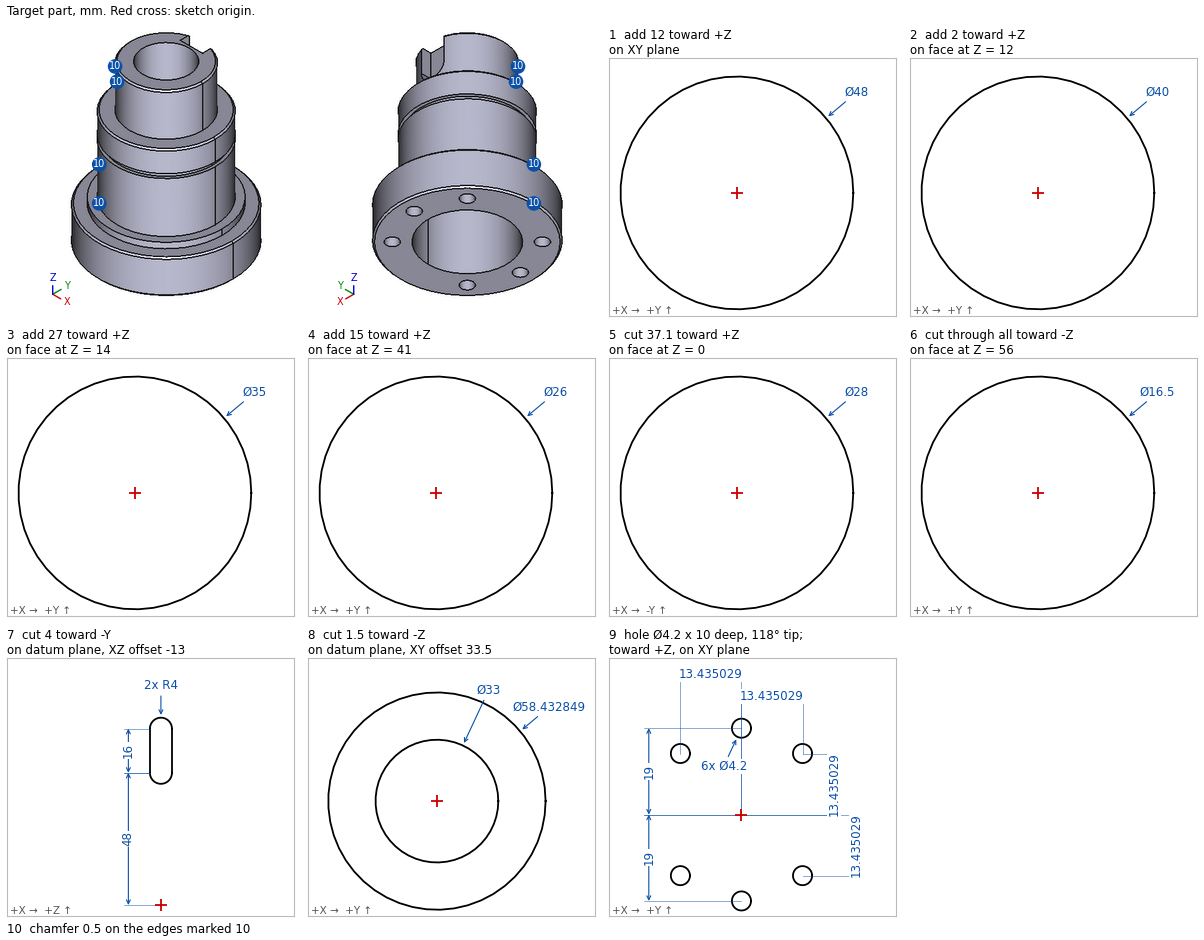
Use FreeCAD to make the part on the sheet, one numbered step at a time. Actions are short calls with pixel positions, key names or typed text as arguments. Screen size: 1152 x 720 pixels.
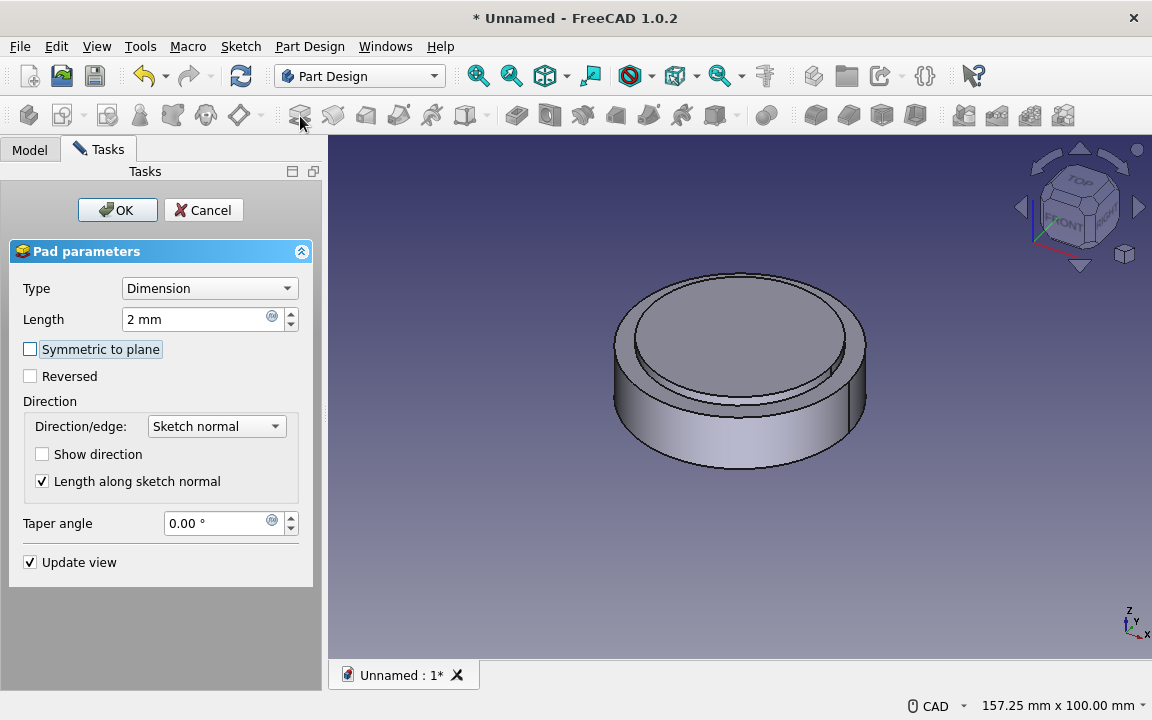
click(118, 210)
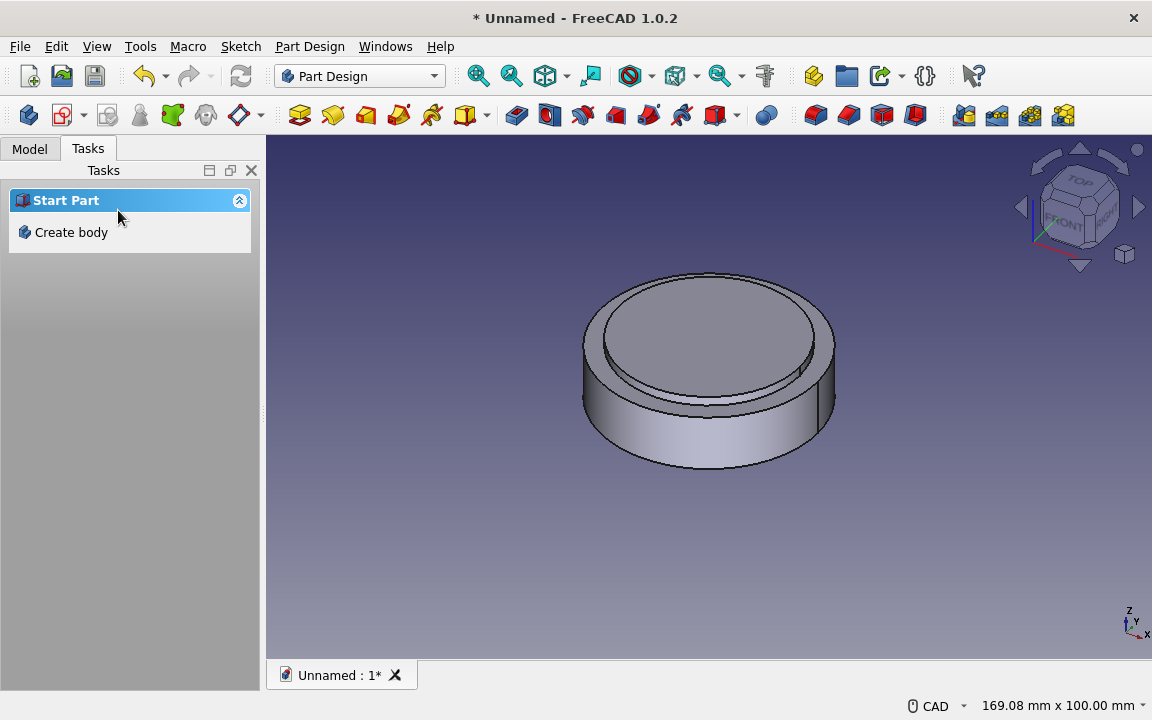
click(709, 336)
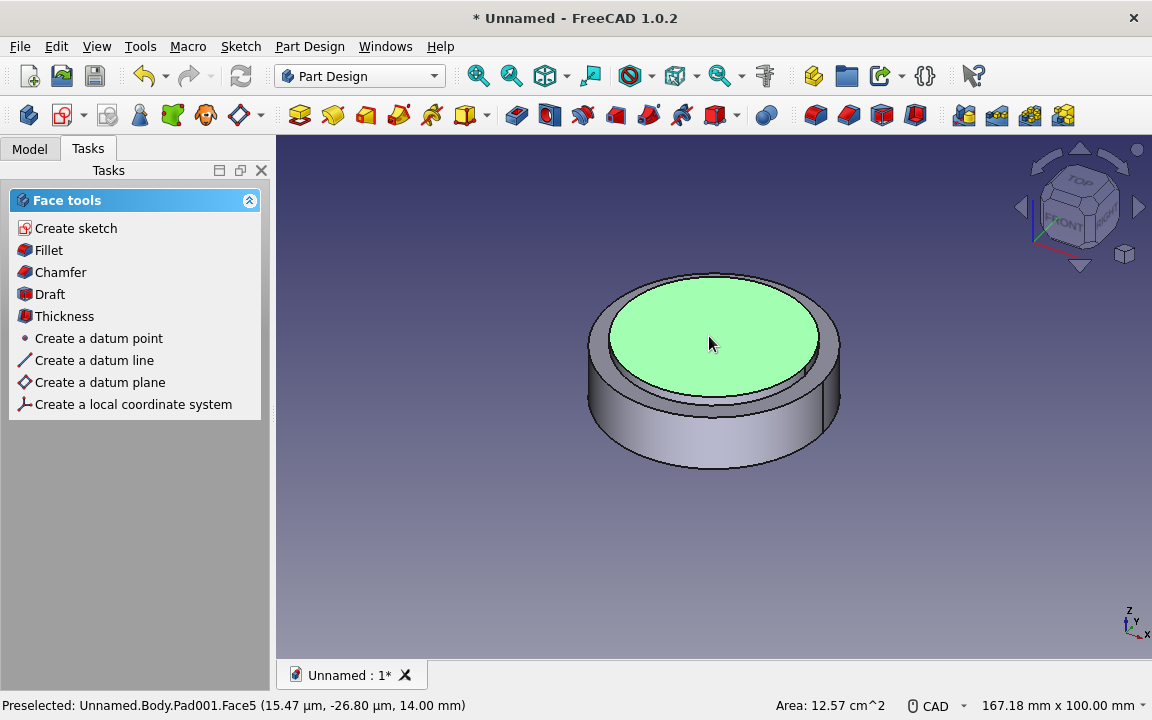
click(62, 116)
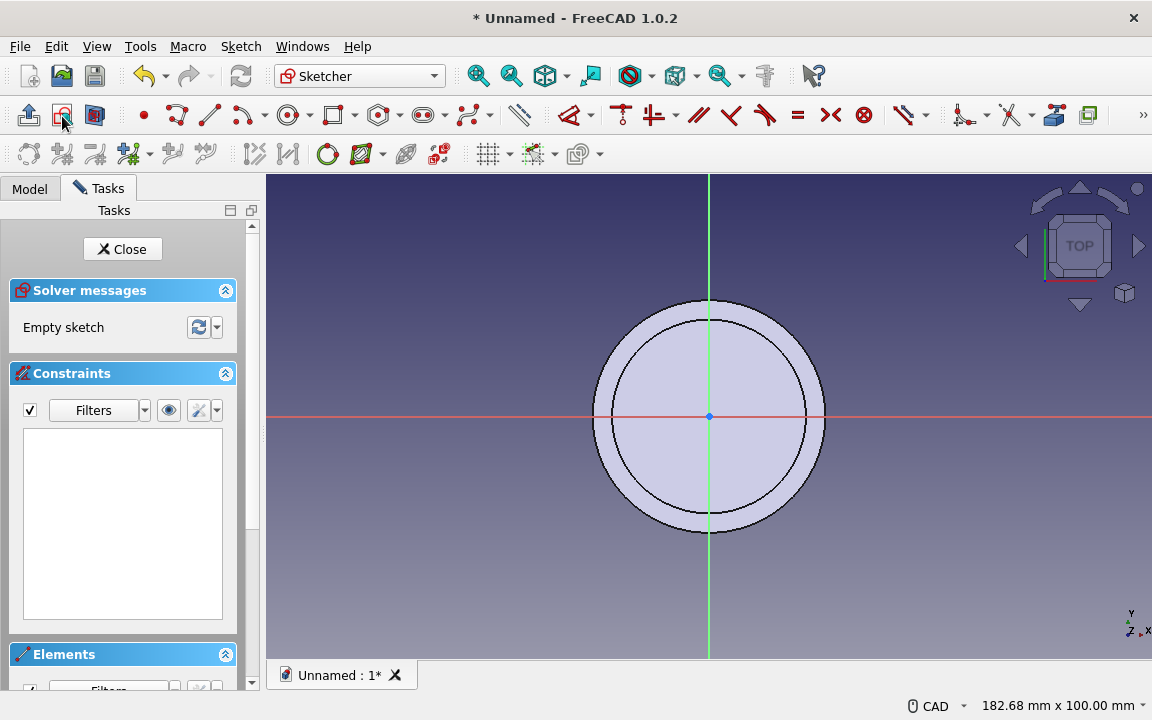
scroll(792, 416, up, 3)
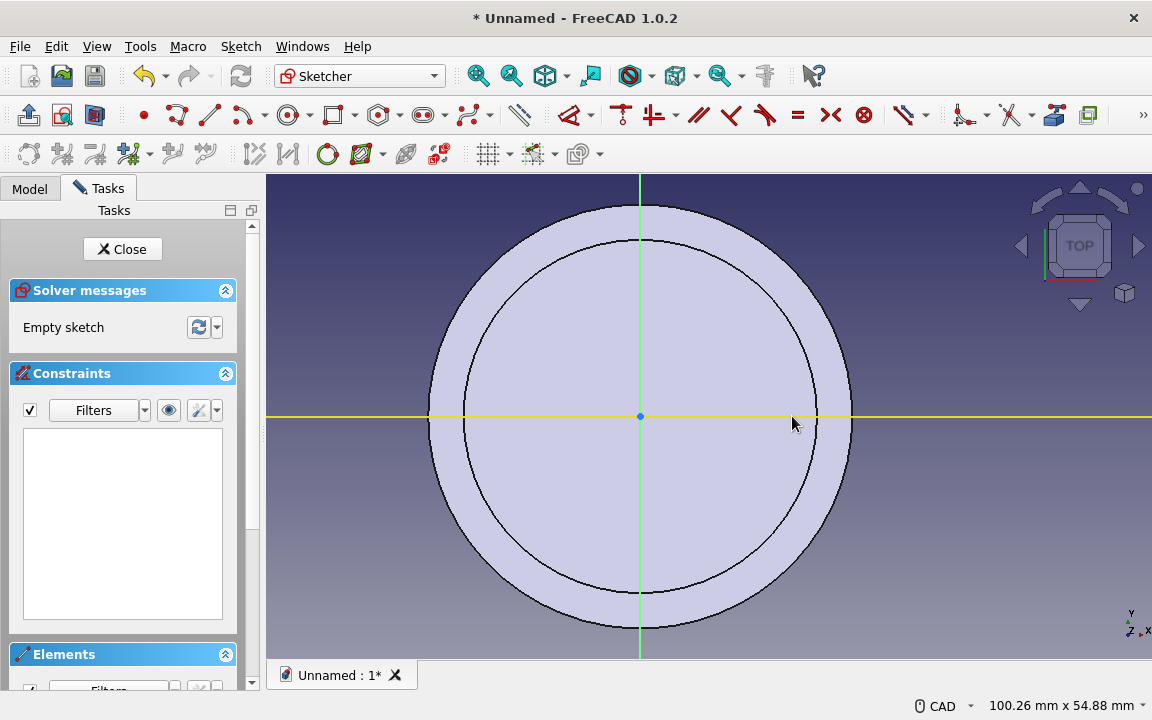
click(288, 116)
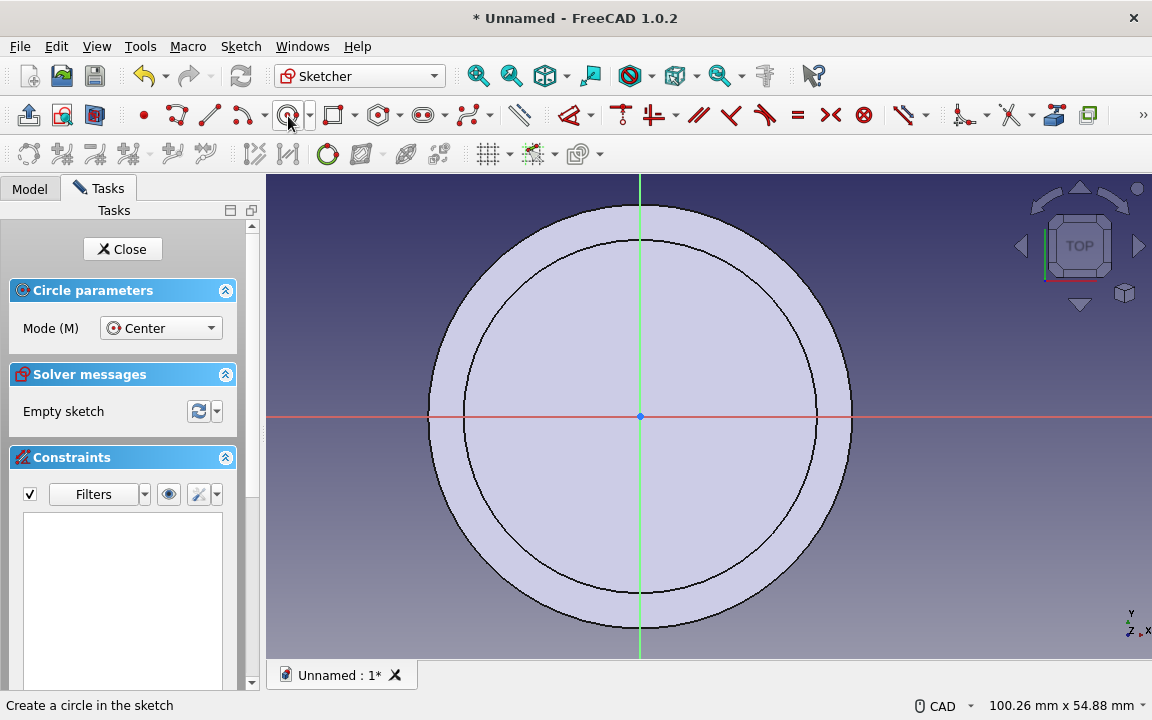
click(640, 416)
click(750, 307)
key(Escape)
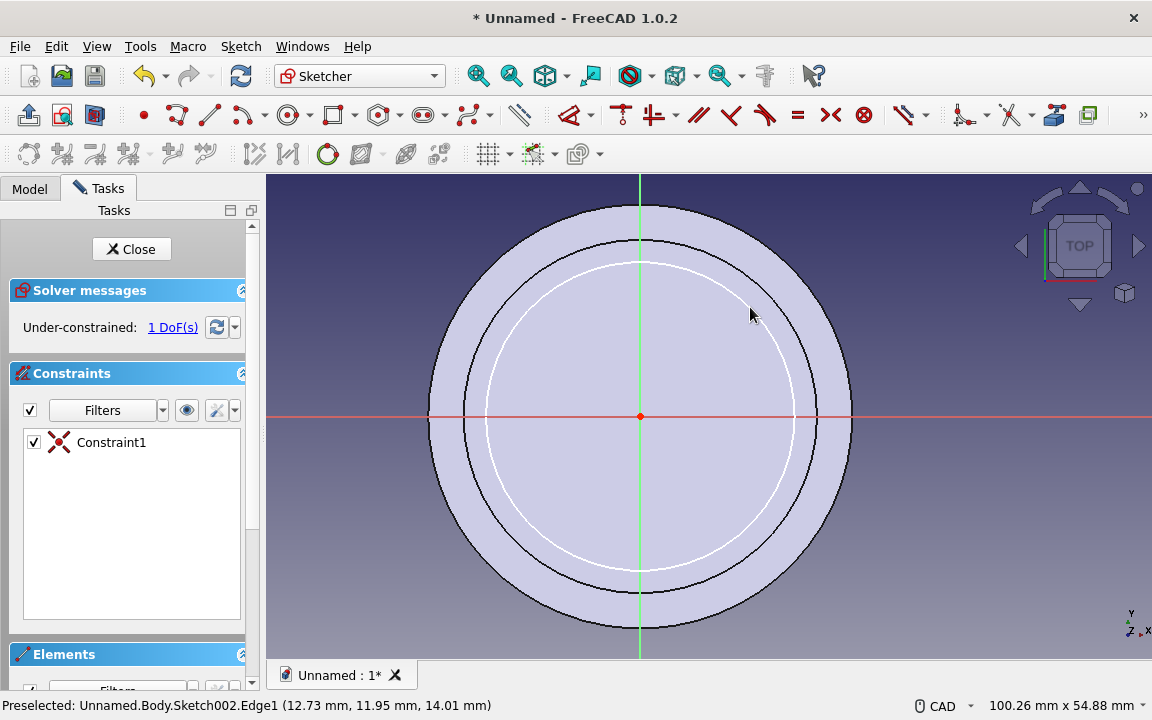
click(749, 307)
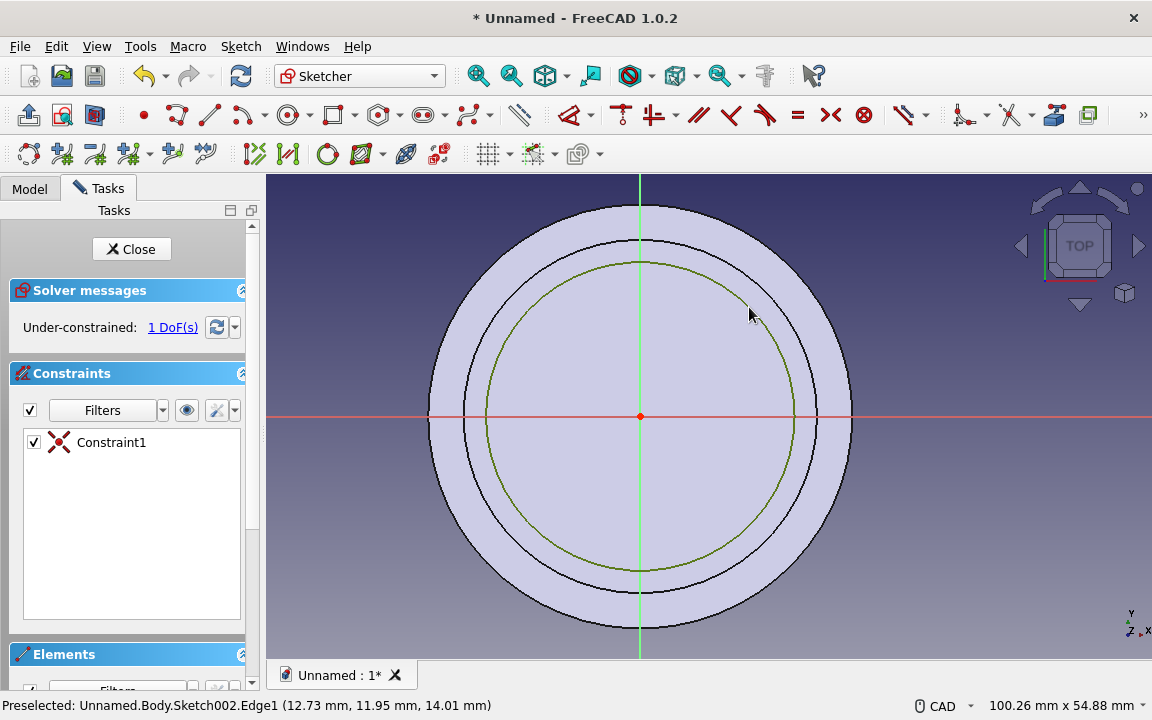
key(k)
key(o)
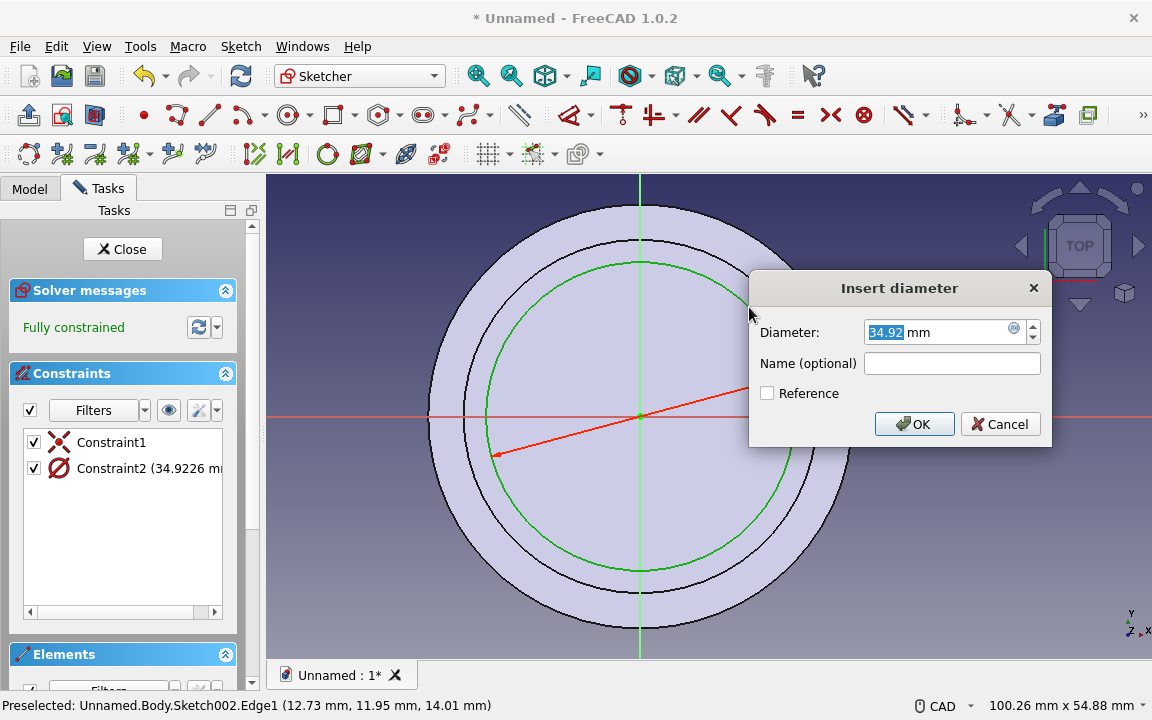
text(35)
key(Return)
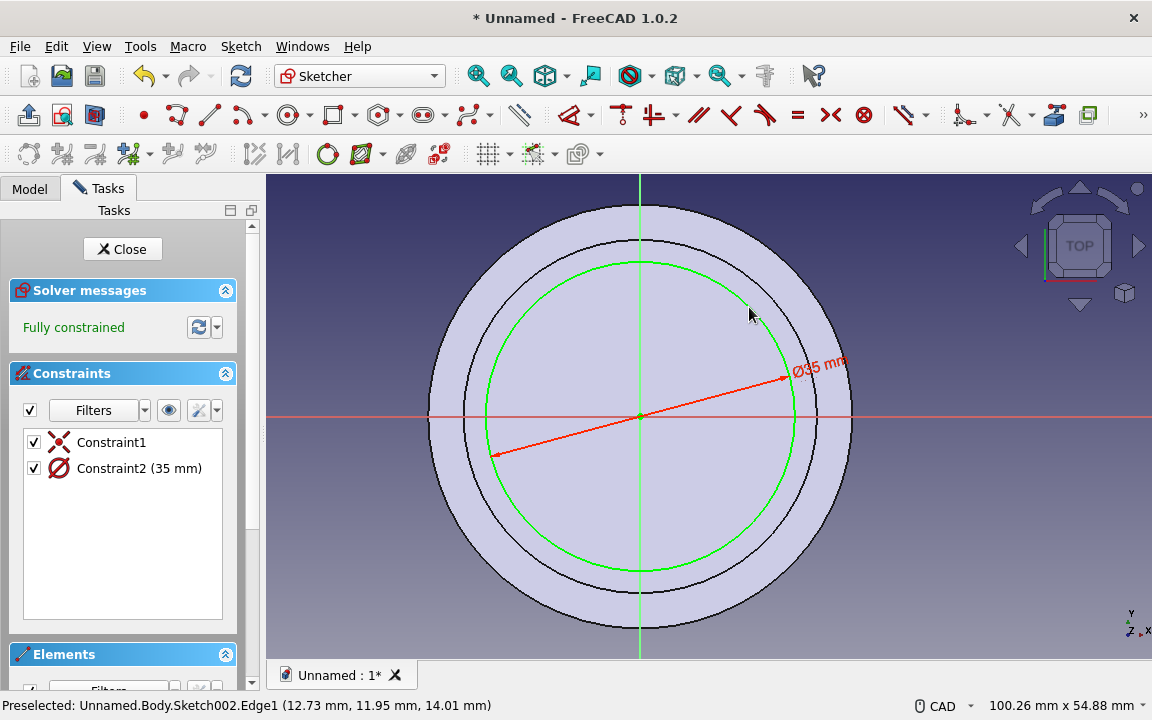
click(123, 249)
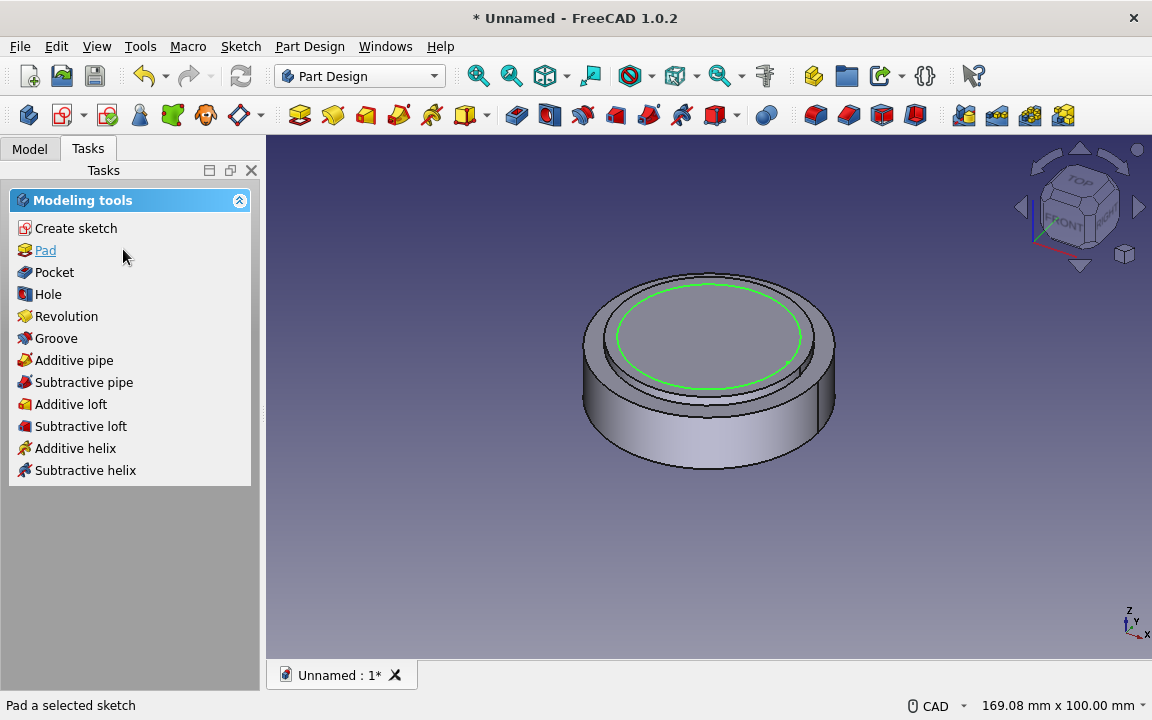
click(300, 116)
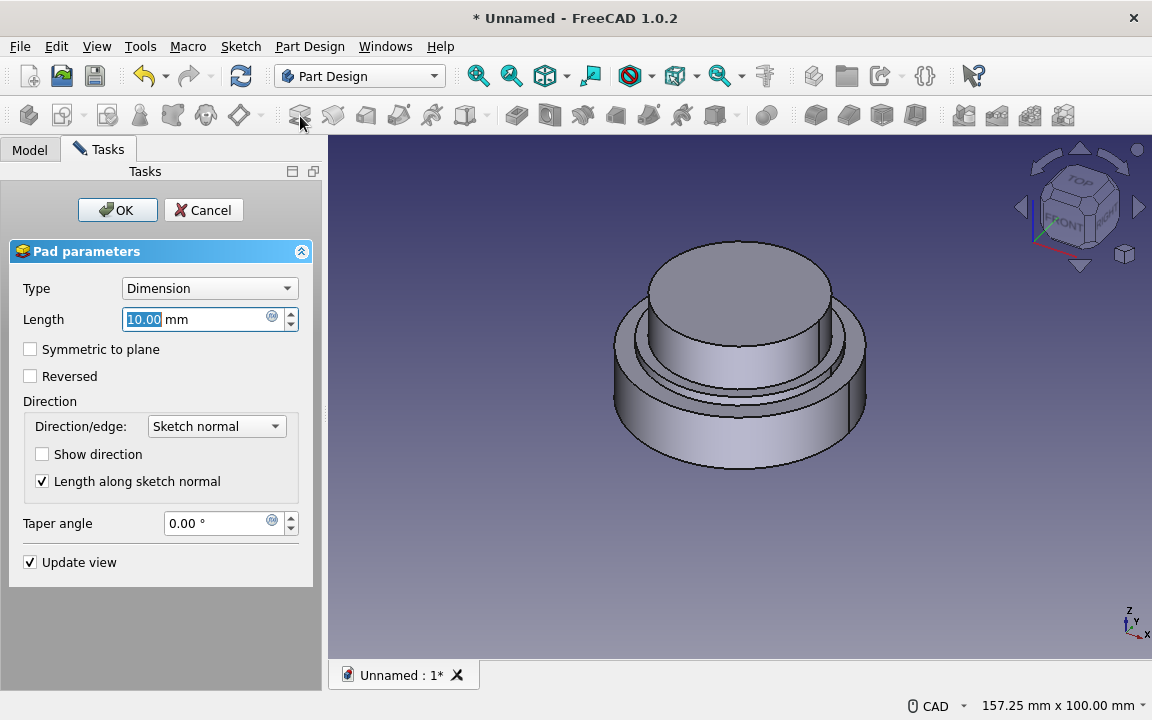
text(27)
key(Tab)